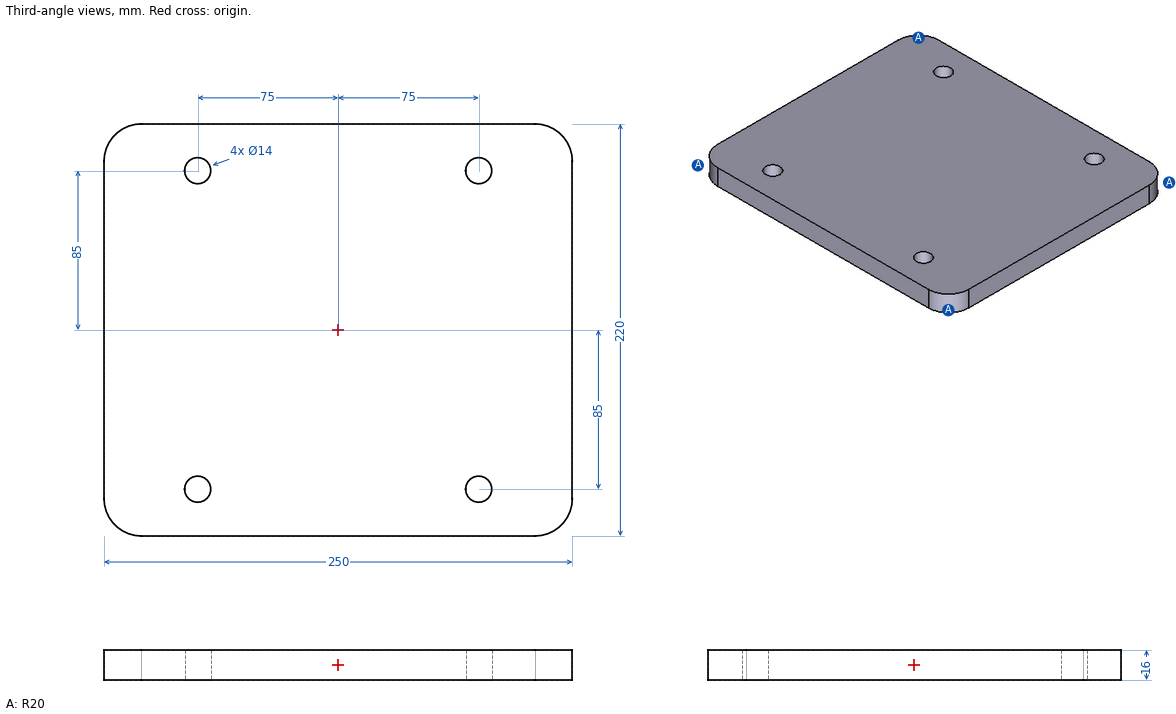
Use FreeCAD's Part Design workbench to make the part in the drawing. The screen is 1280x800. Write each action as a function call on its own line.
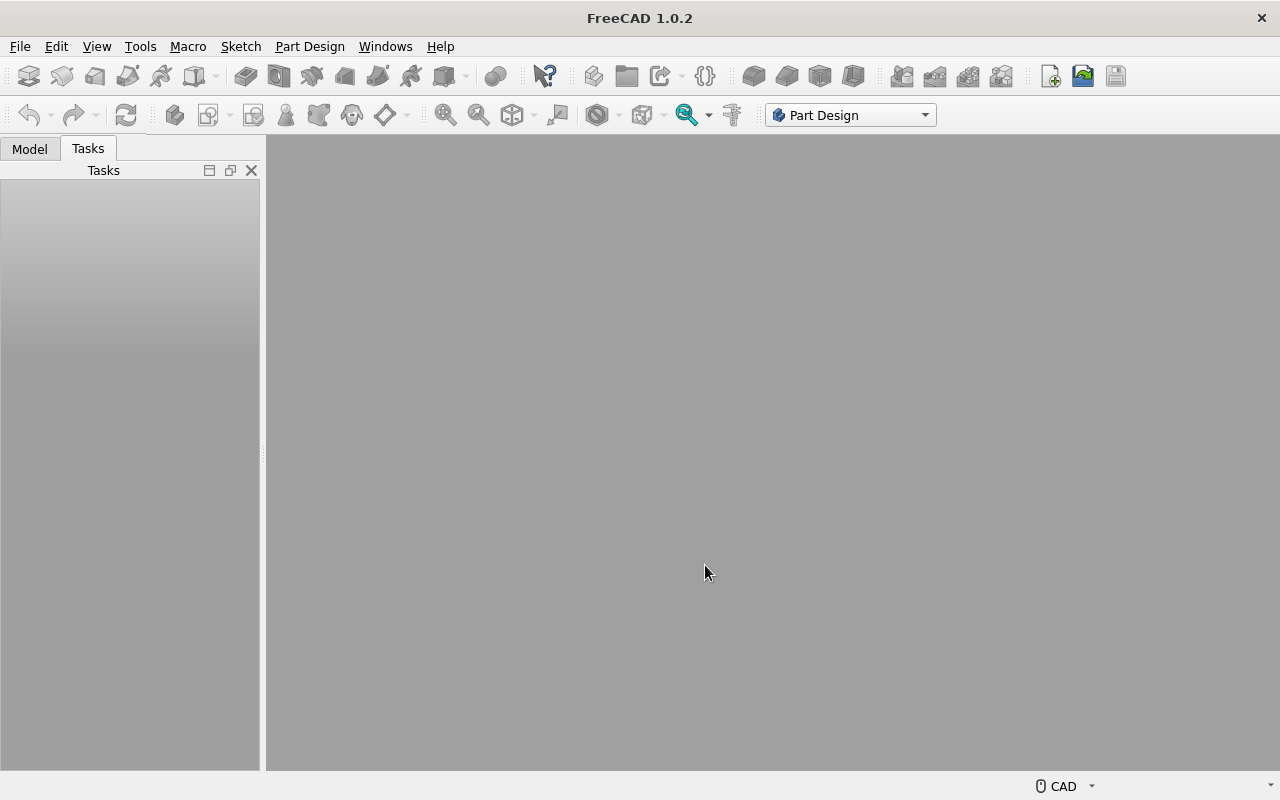
click(1050, 76)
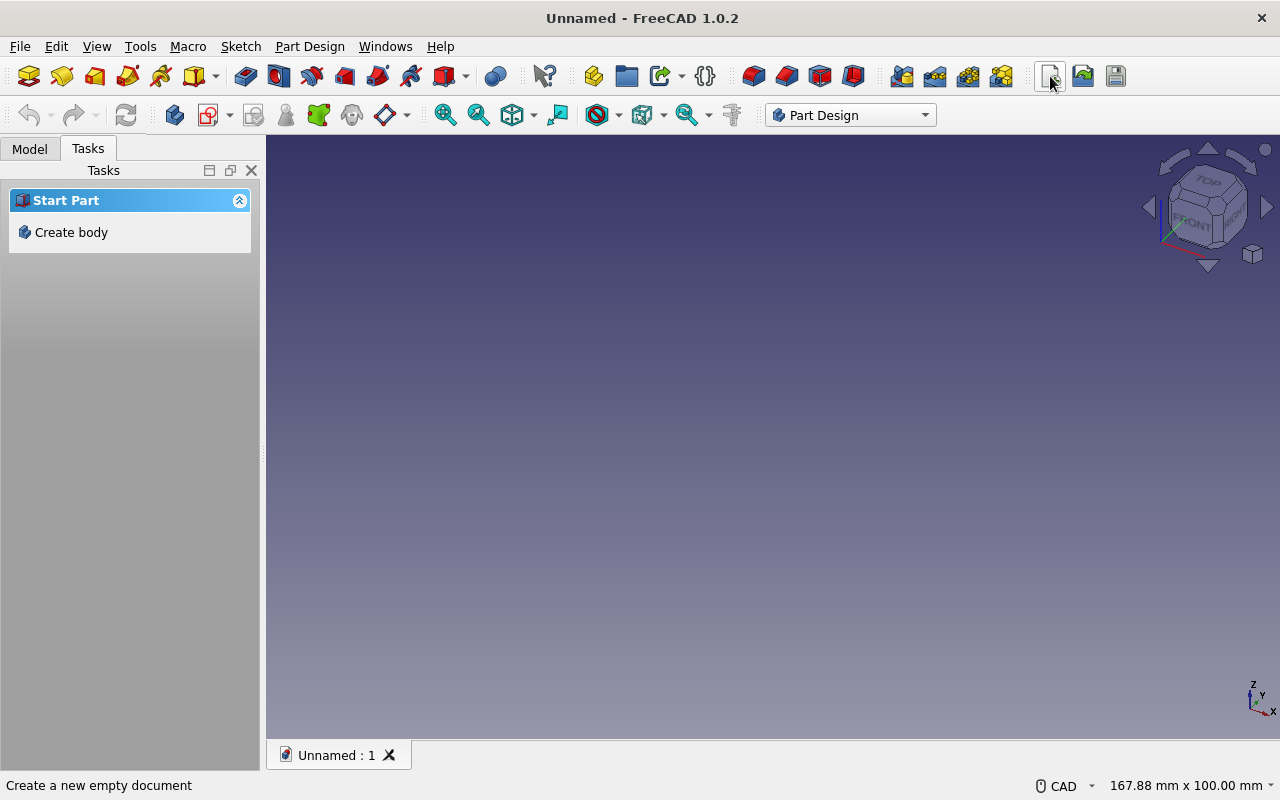
click(208, 116)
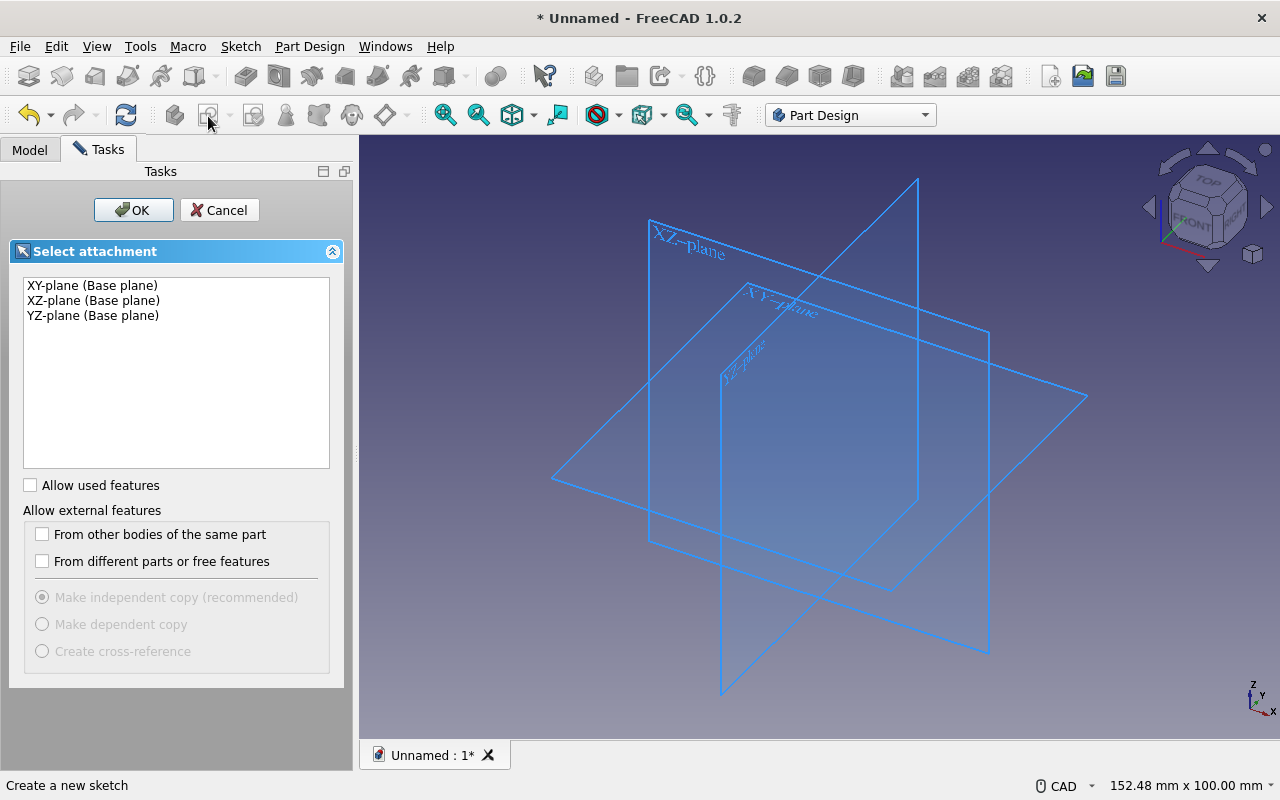
click(84, 286)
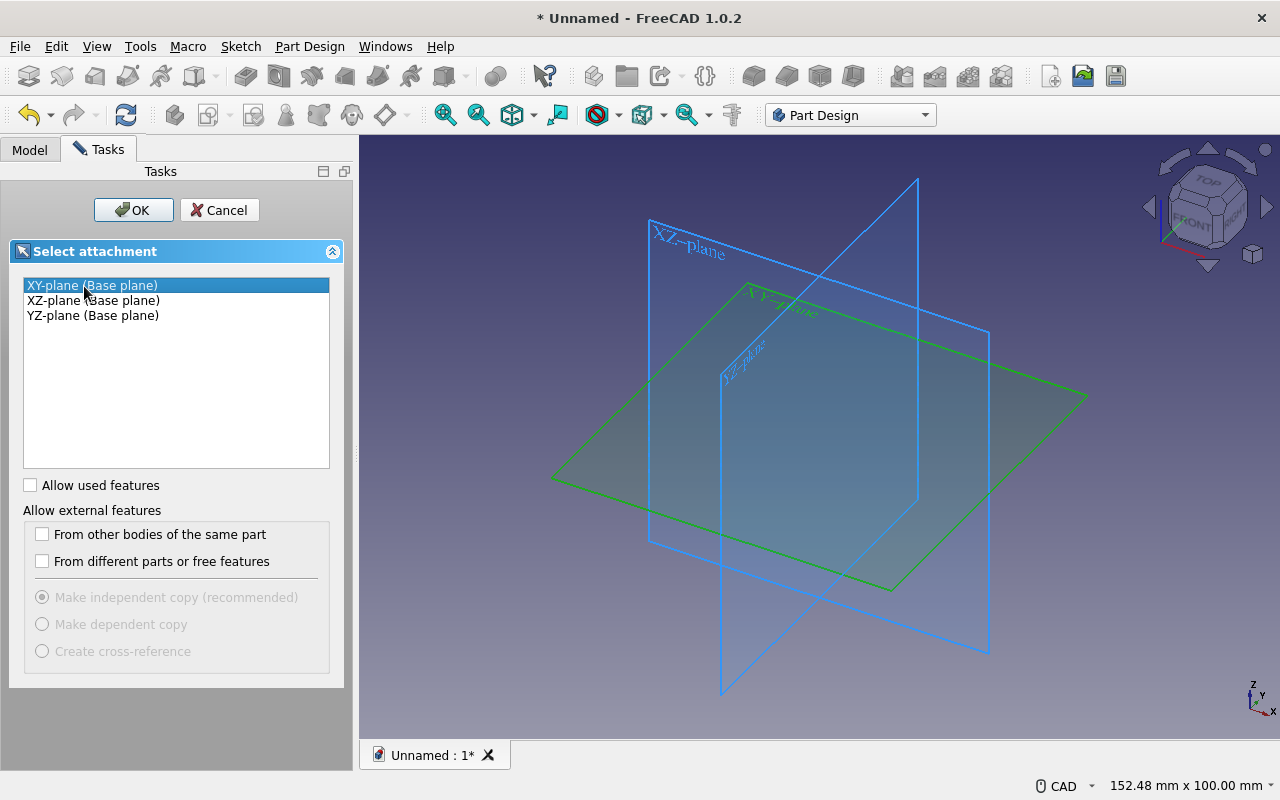
click(134, 210)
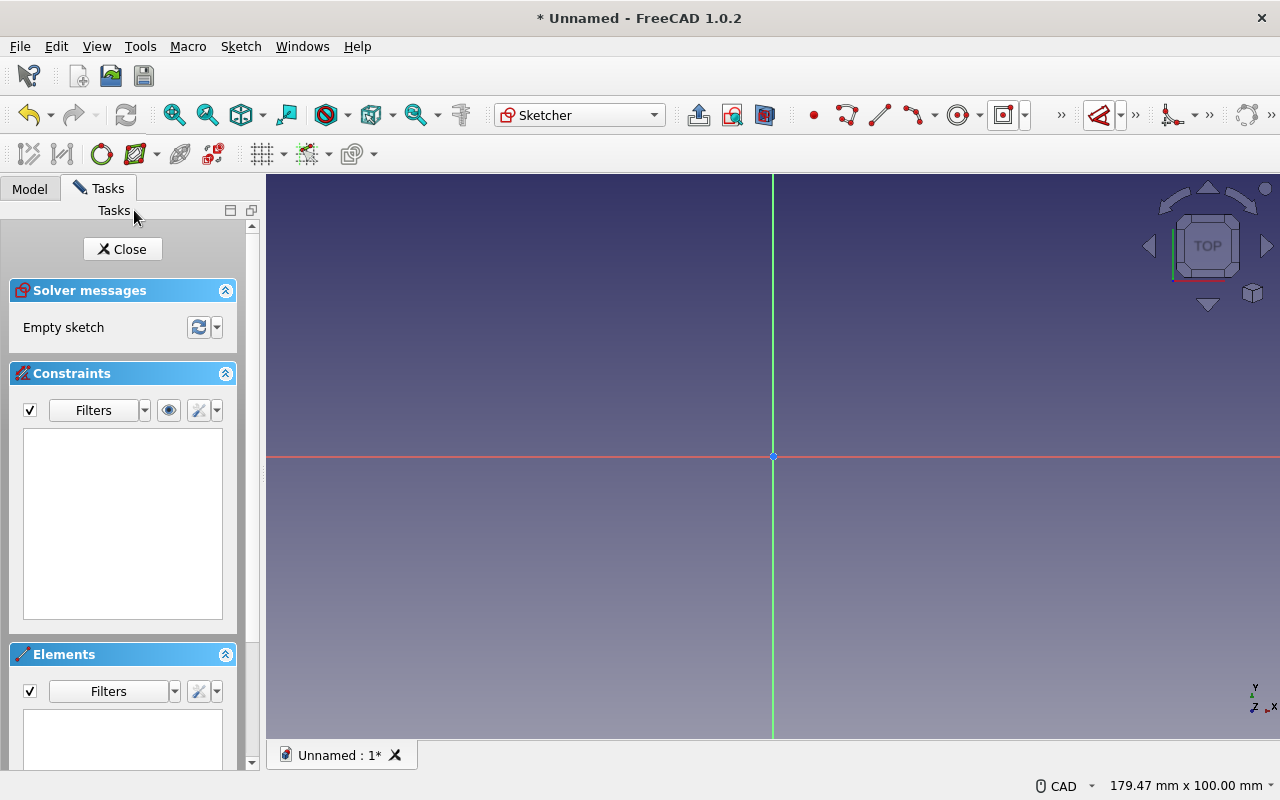
scroll(675, 456, down, 6)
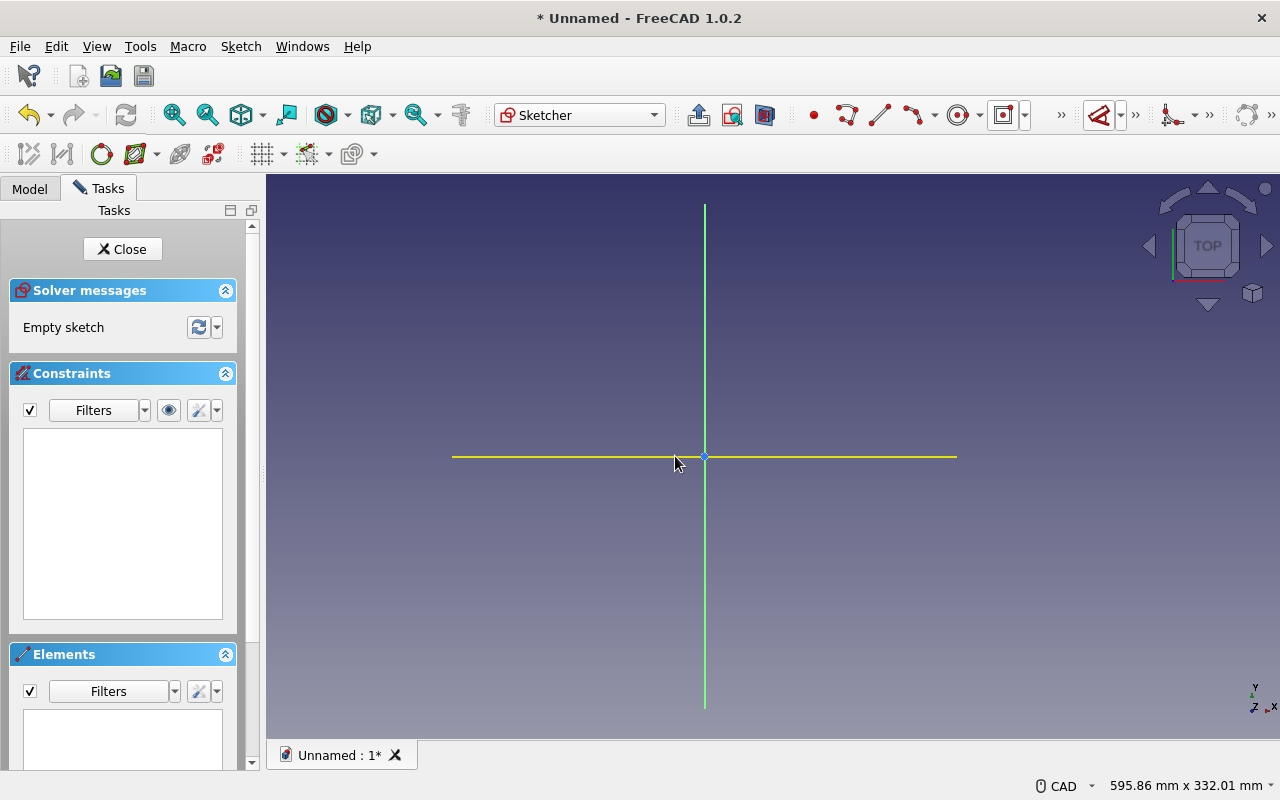
click(1002, 116)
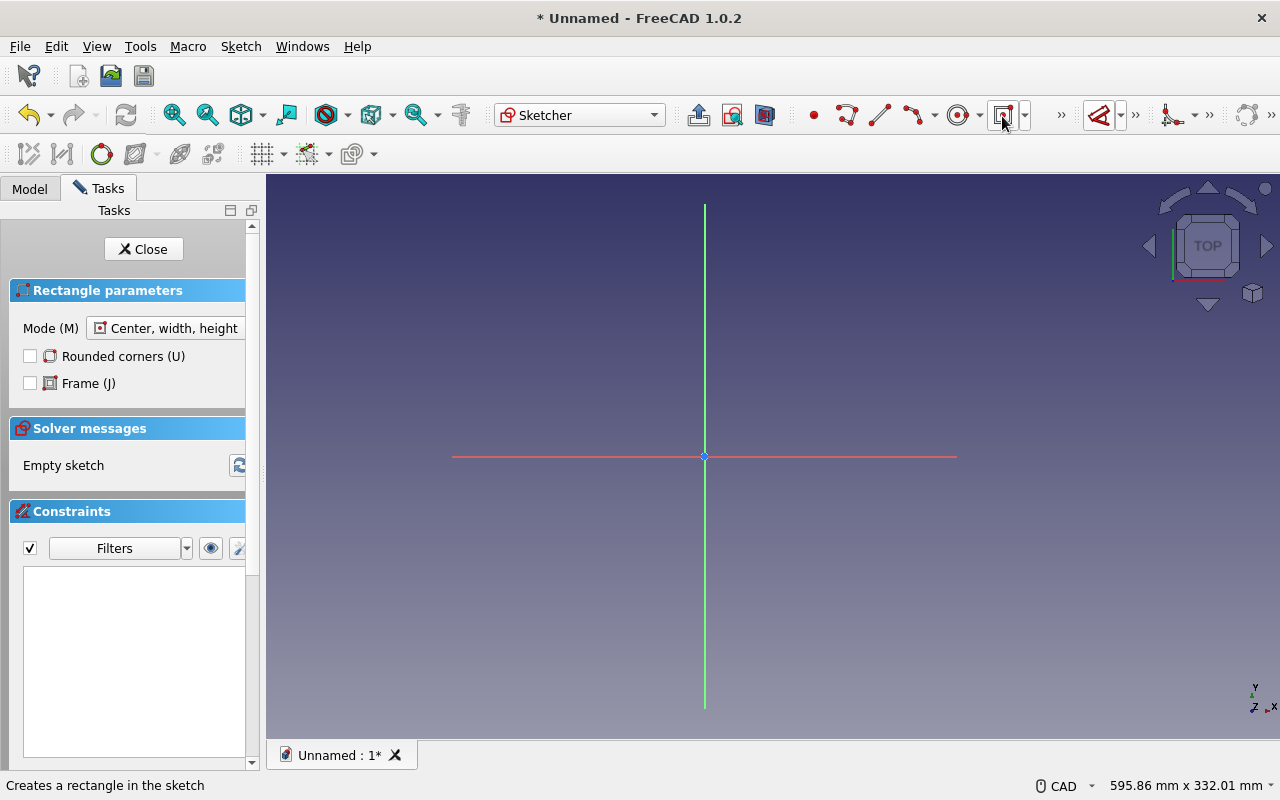
click(705, 456)
move(918, 269)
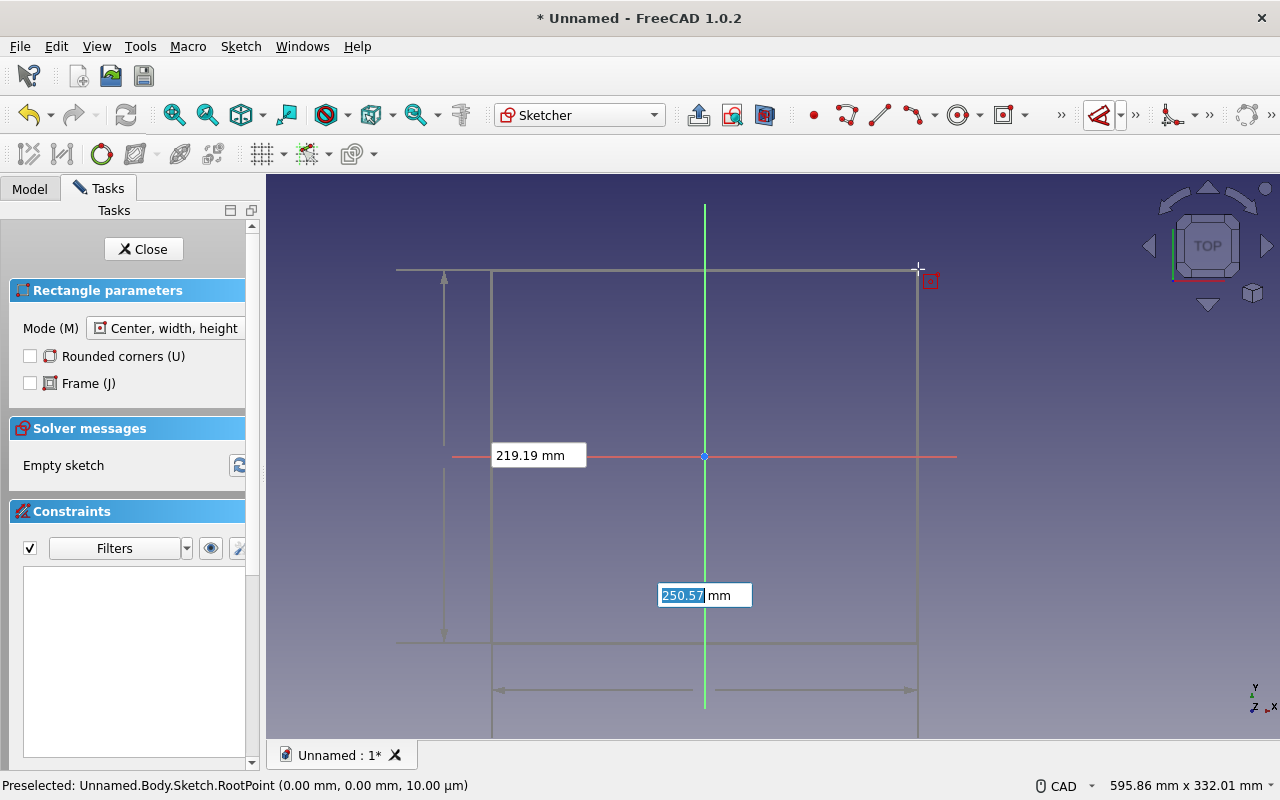
text(250)
key(Tab)
text(220)
key(Return)
key(Escape)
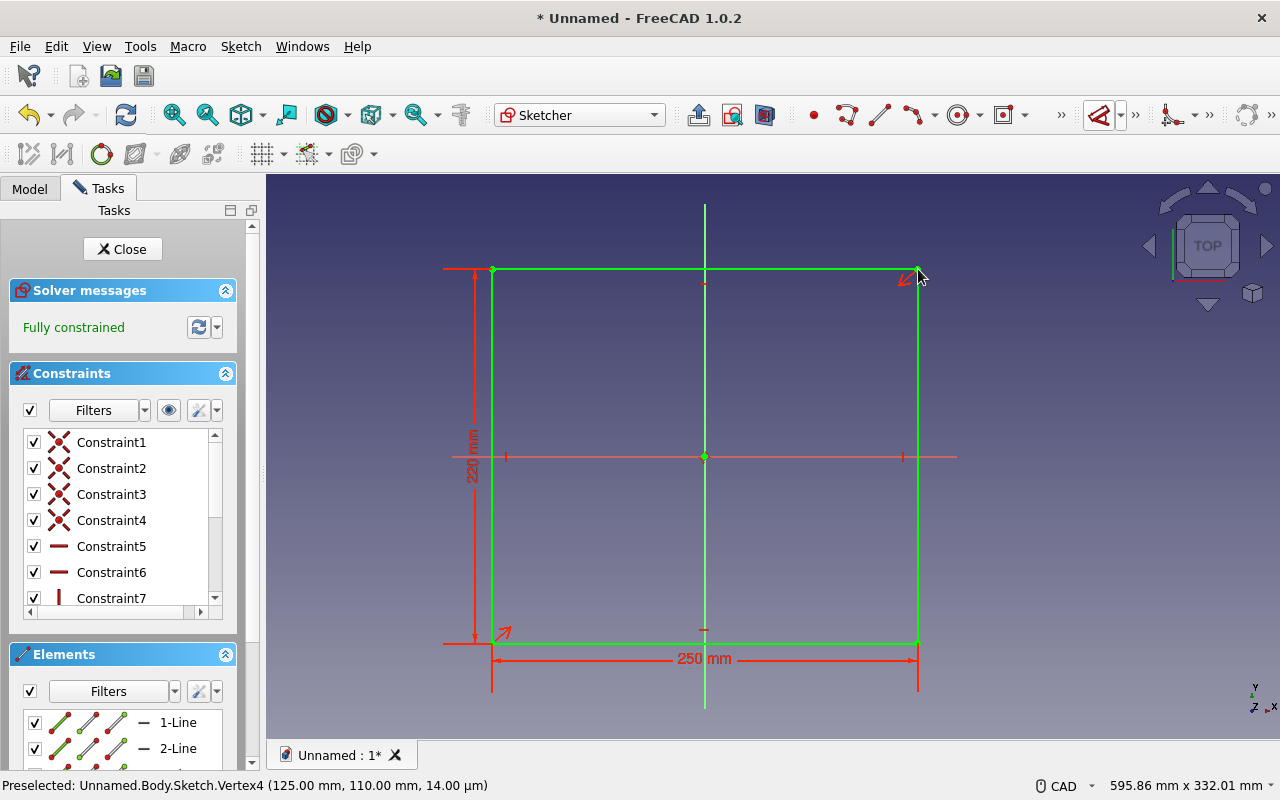
click(123, 249)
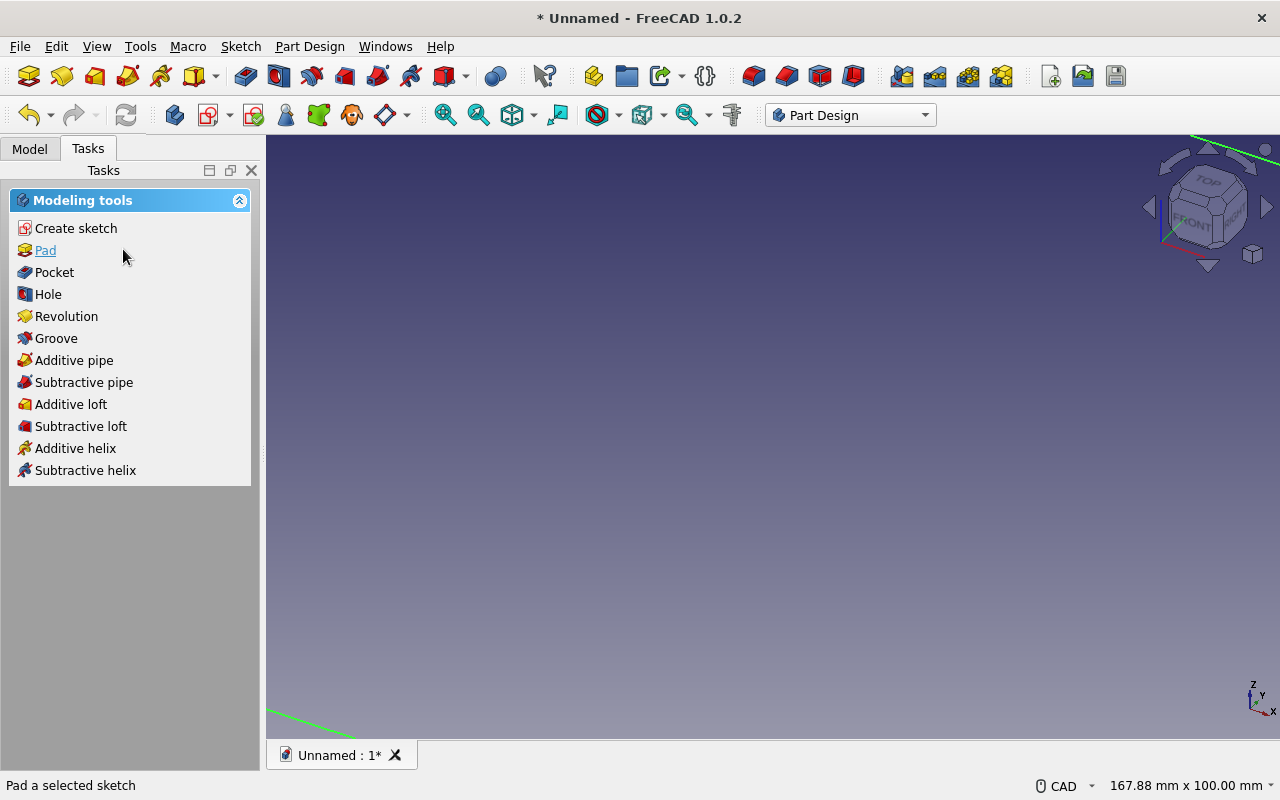
click(29, 76)